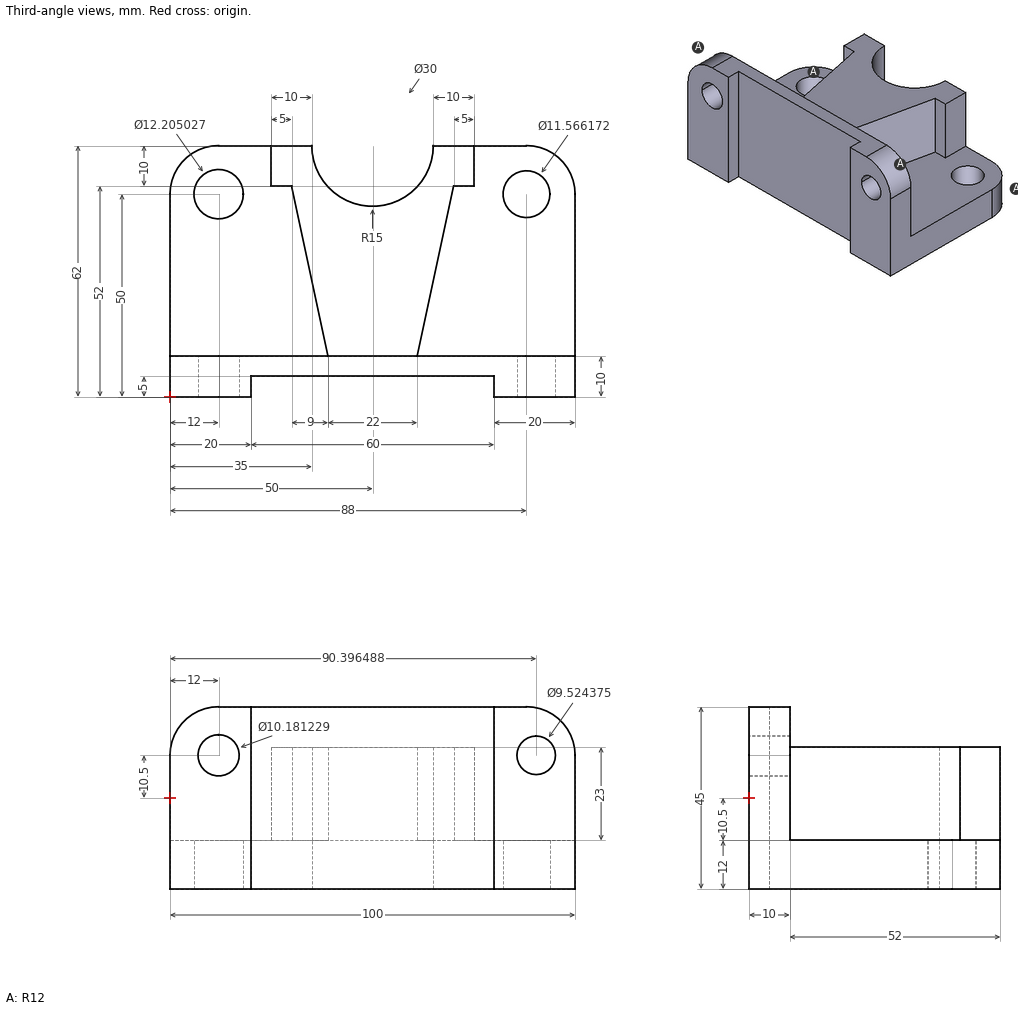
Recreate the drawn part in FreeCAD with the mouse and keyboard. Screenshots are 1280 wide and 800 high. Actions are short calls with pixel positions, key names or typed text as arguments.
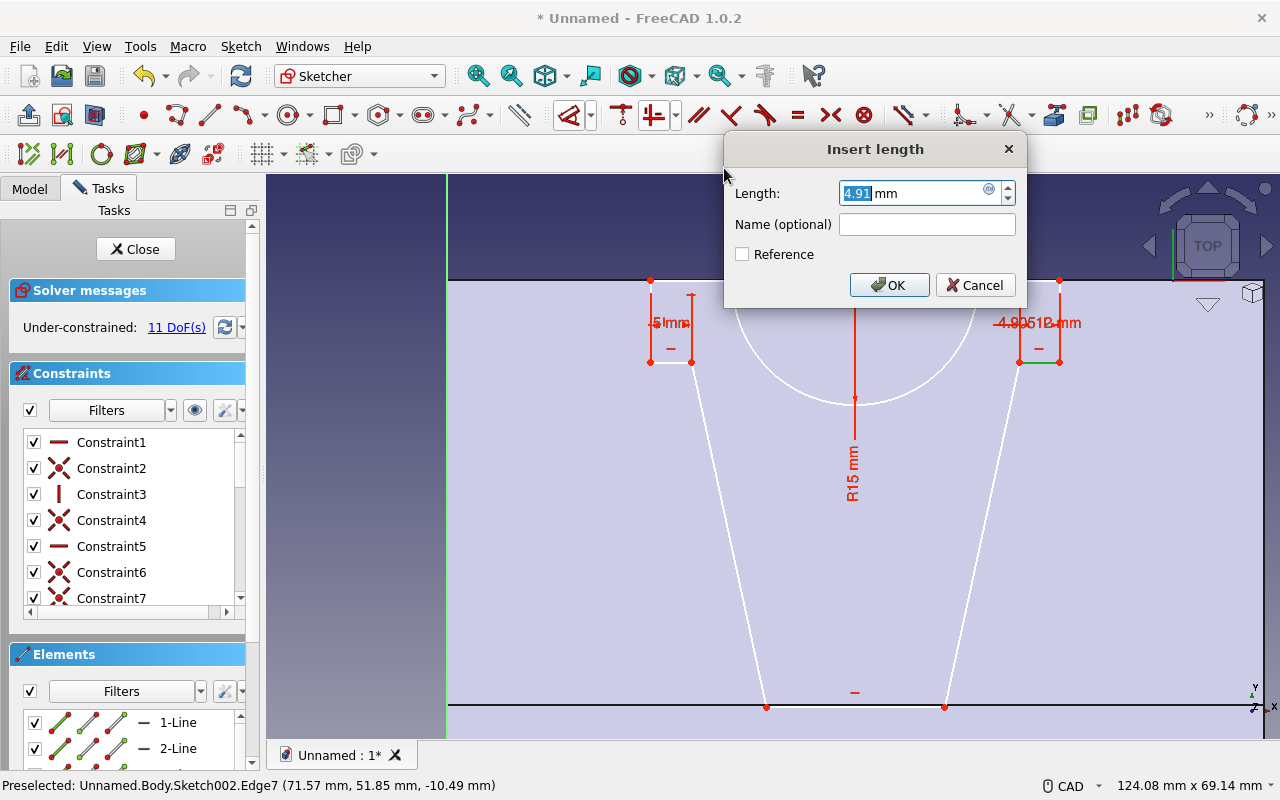
text(5)
key(Return)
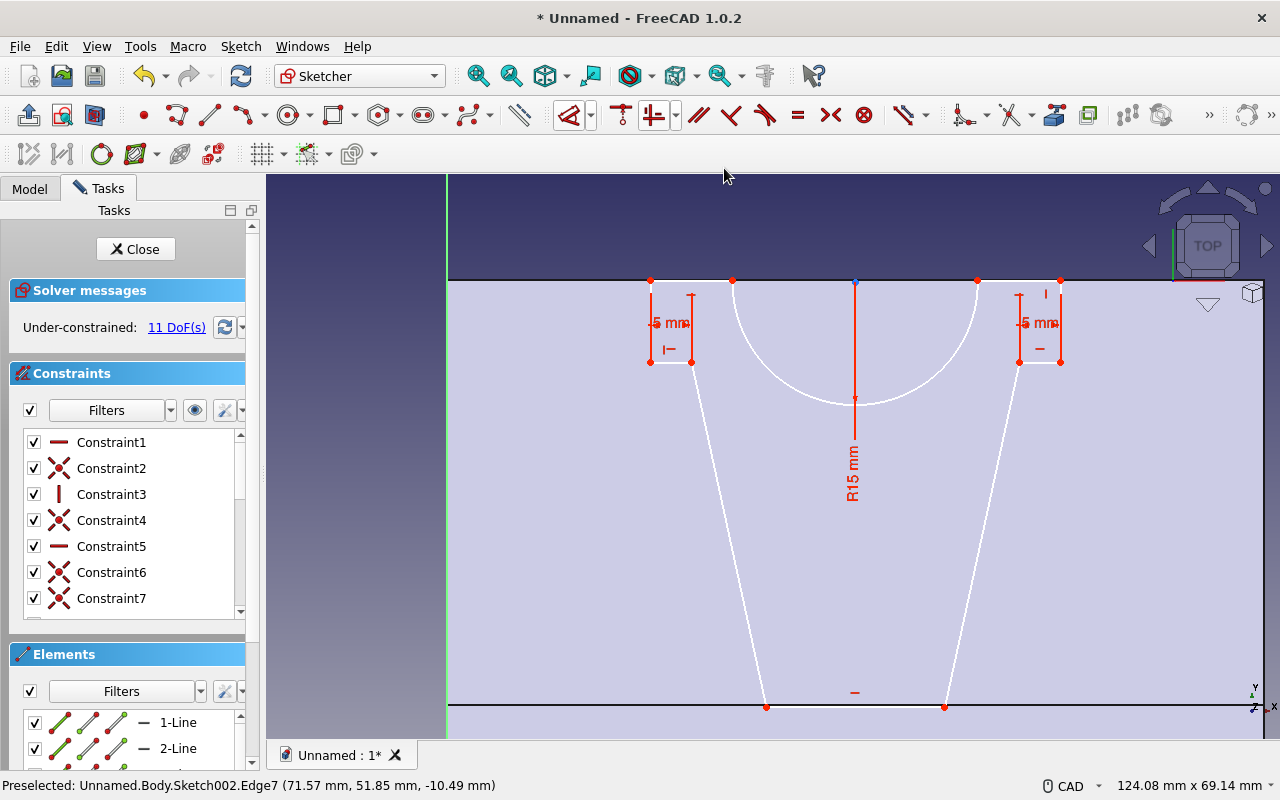
click(708, 281)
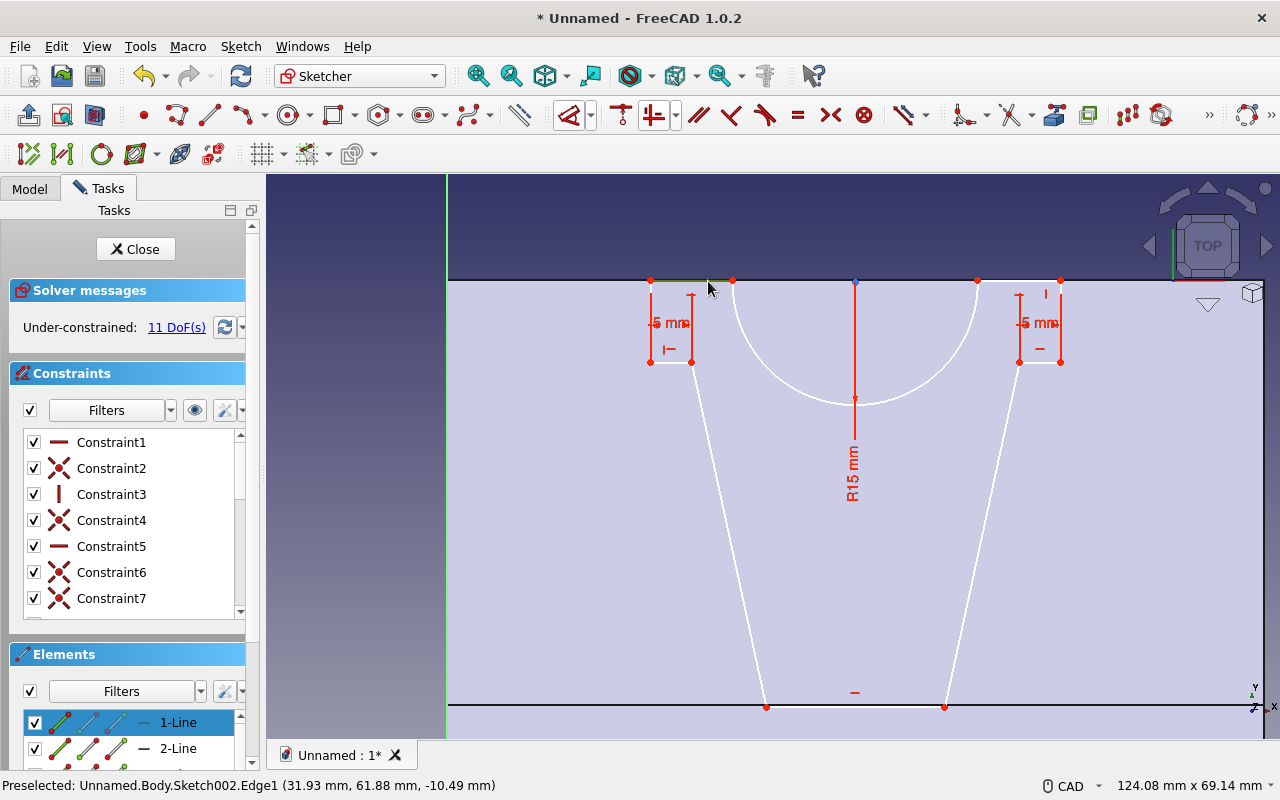
key(l)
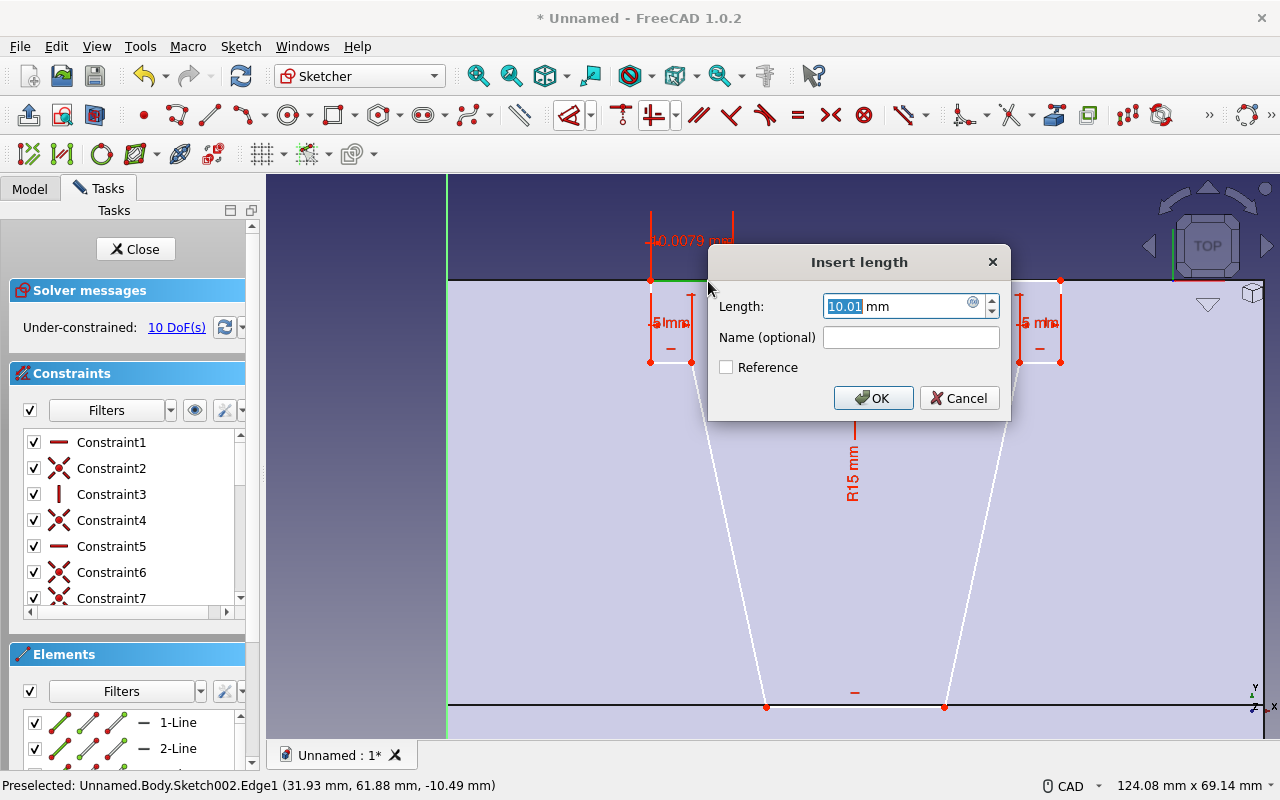
text(10)
key(Return)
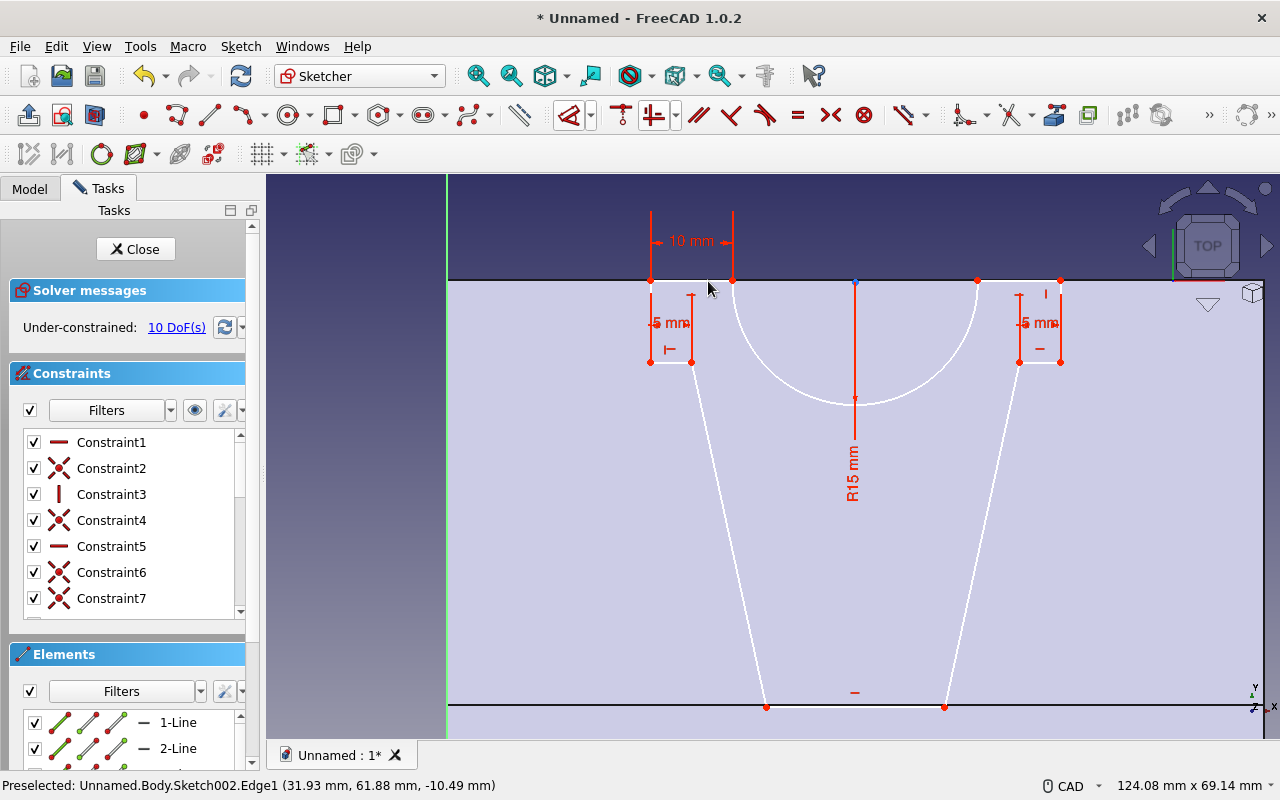
click(651, 305)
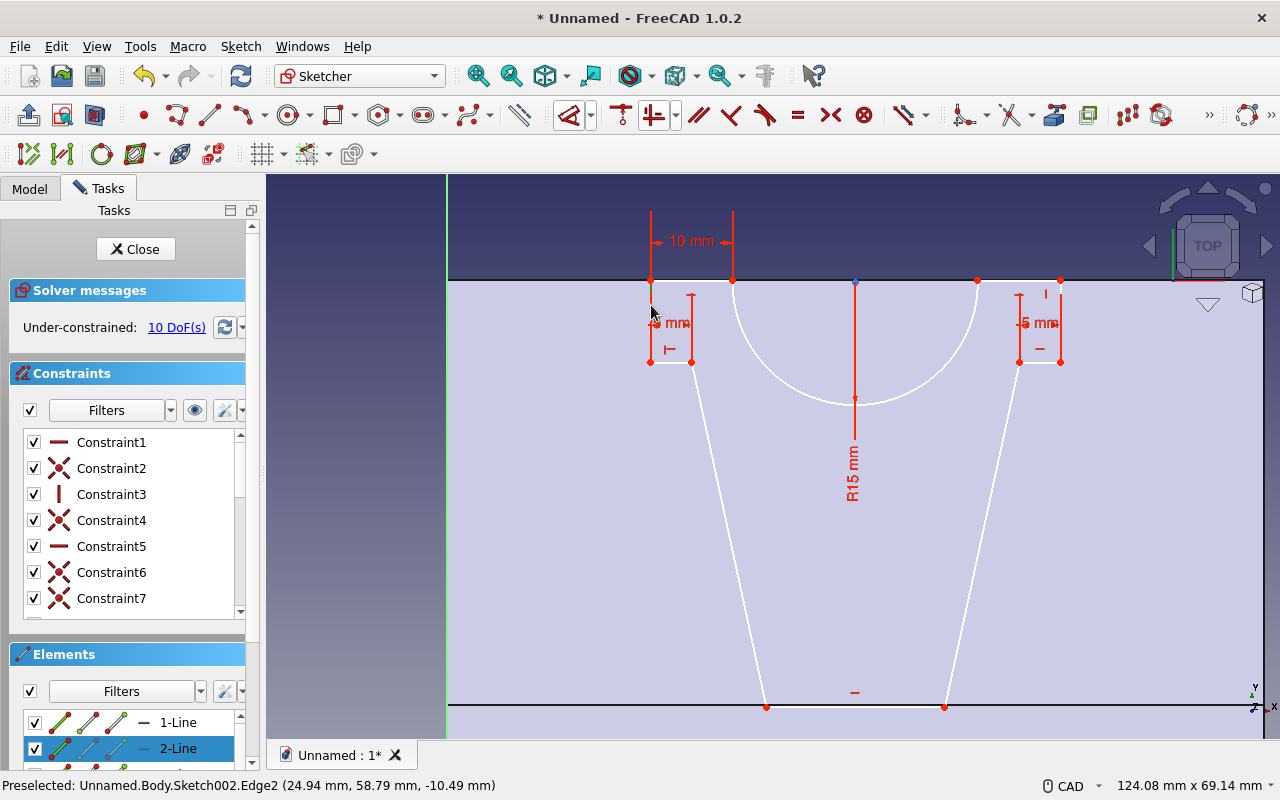
key(i)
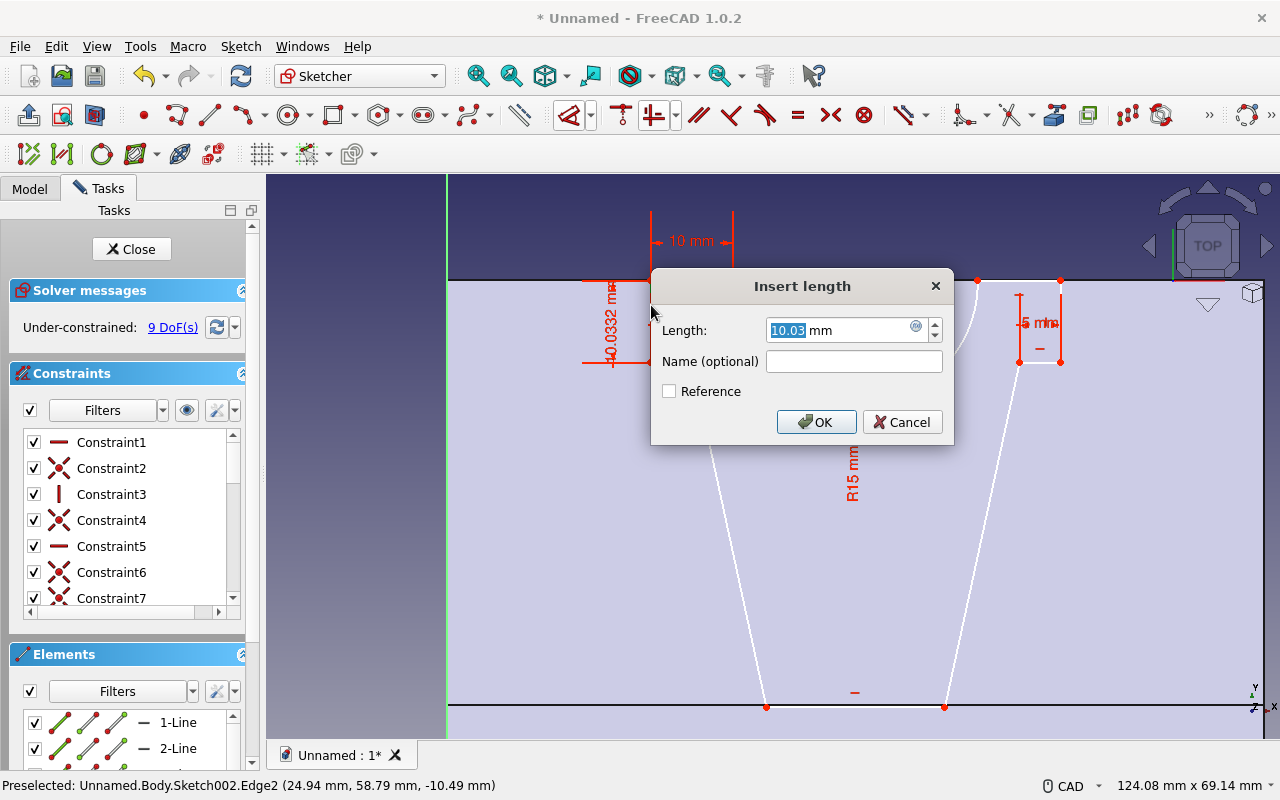
text(10)
key(Return)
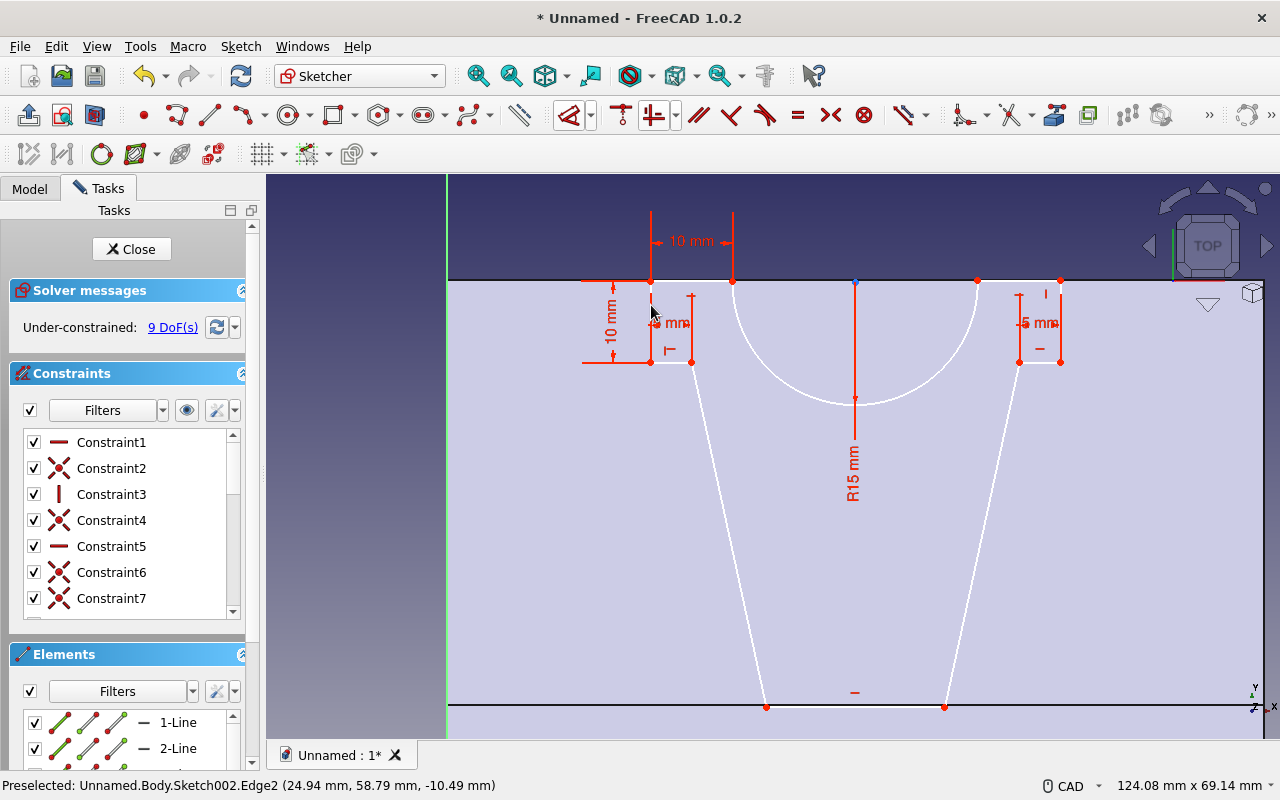
click(820, 707)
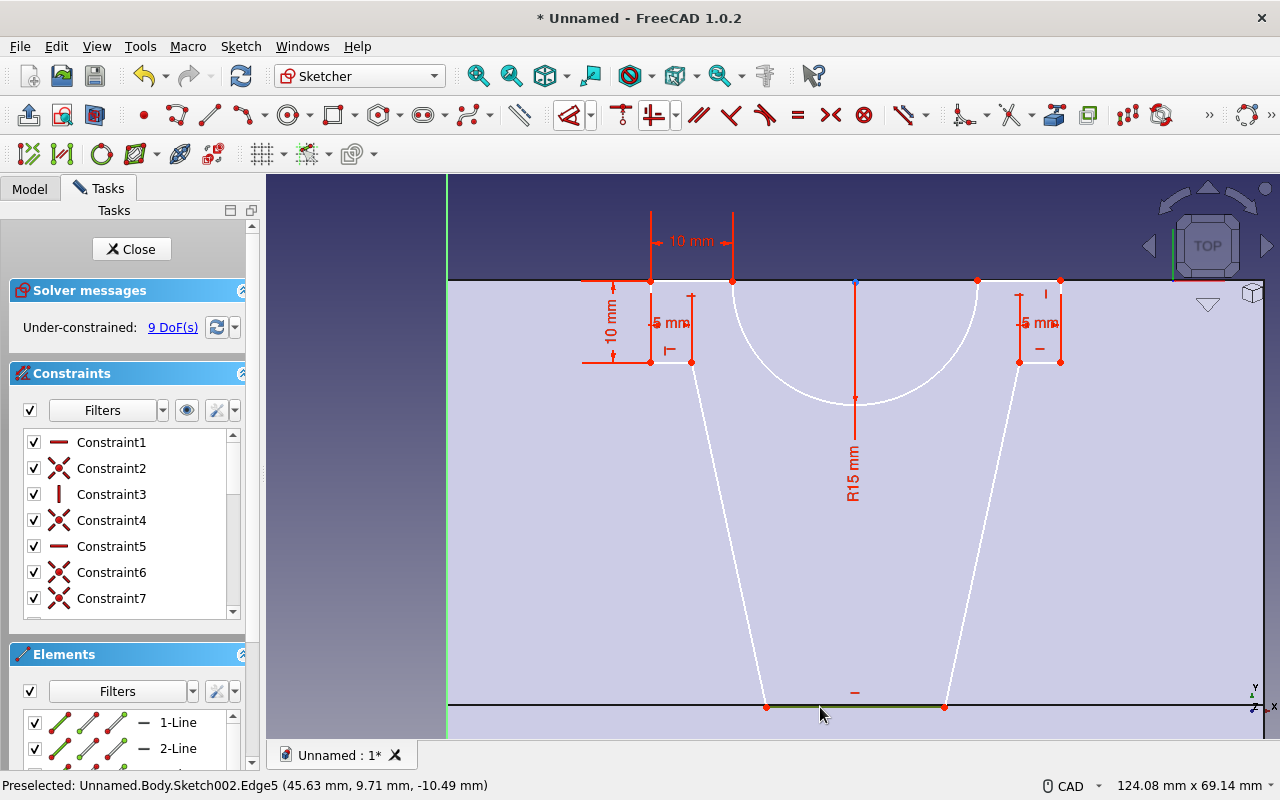
key(l)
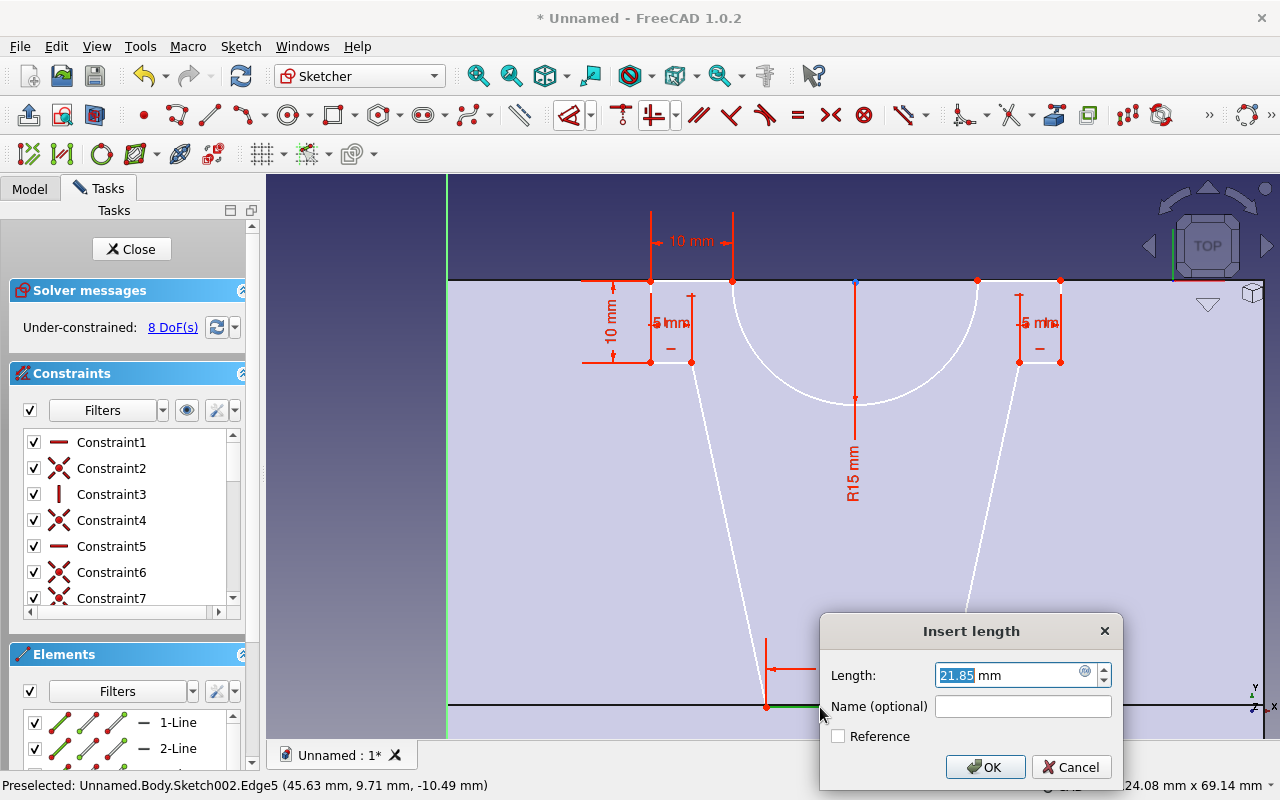
text(22)
key(Return)